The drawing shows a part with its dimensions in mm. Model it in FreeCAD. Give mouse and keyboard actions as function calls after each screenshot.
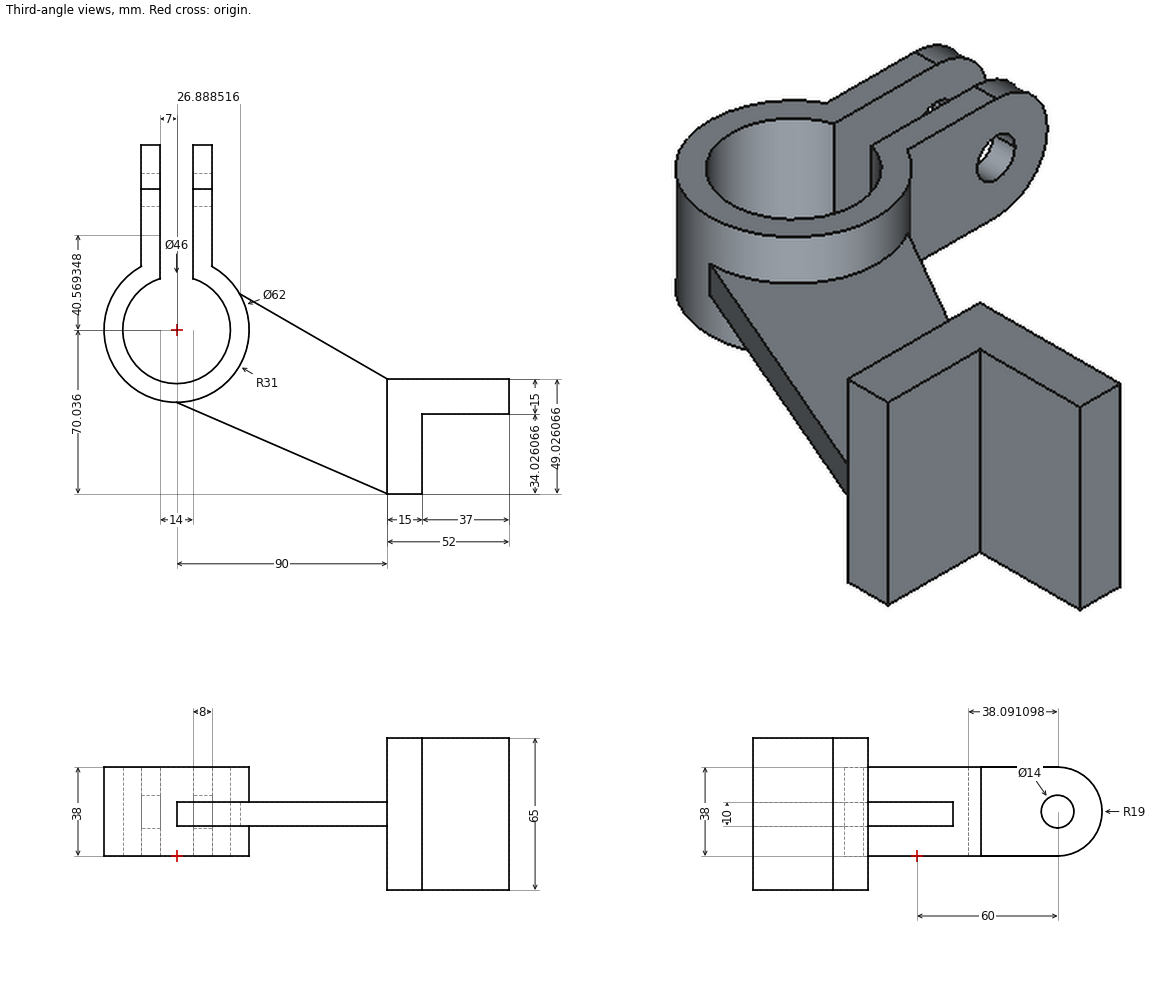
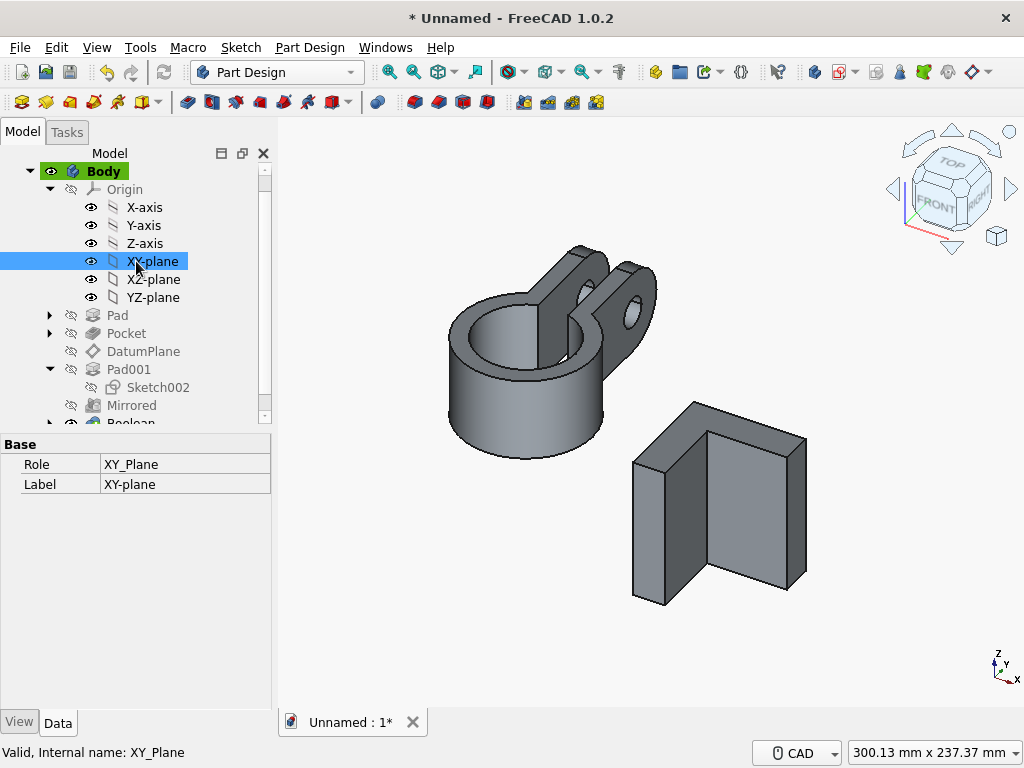
click(972, 72)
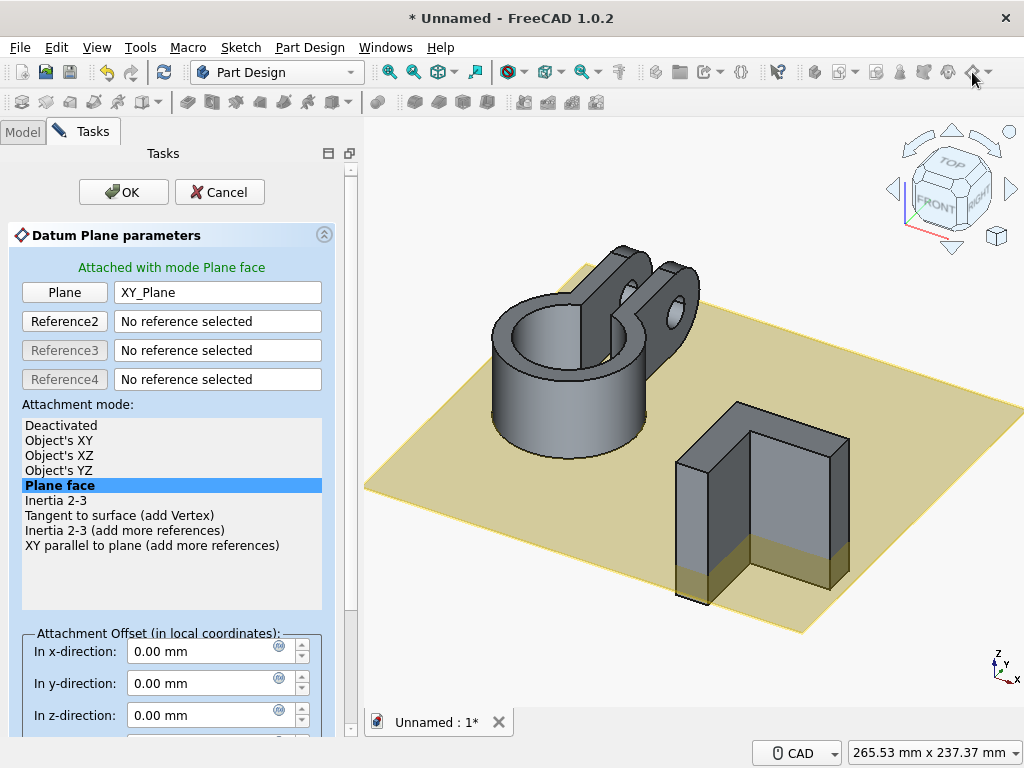
triple_click(210, 715)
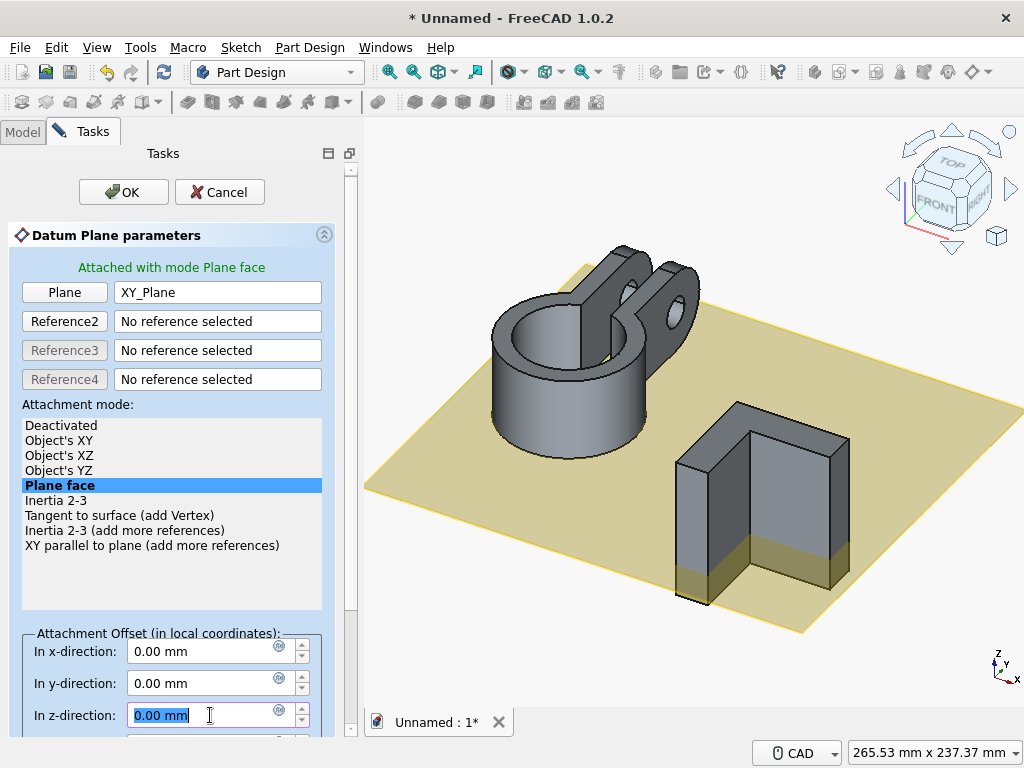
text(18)
key(Tab)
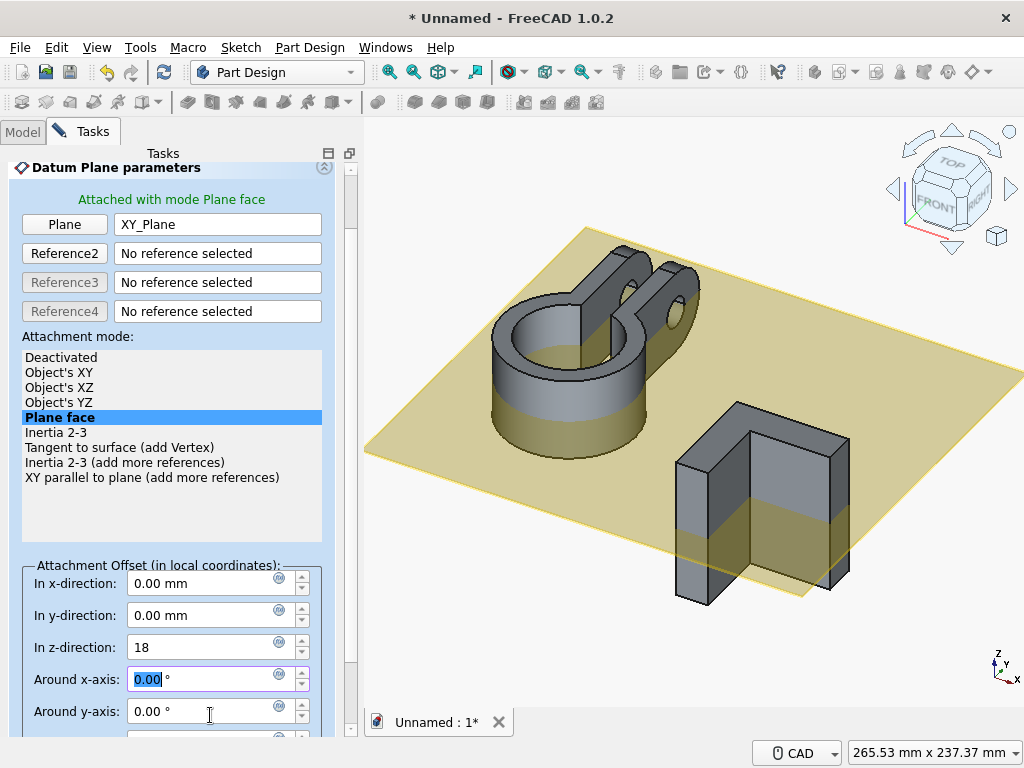
scroll(351, 450, up, 2)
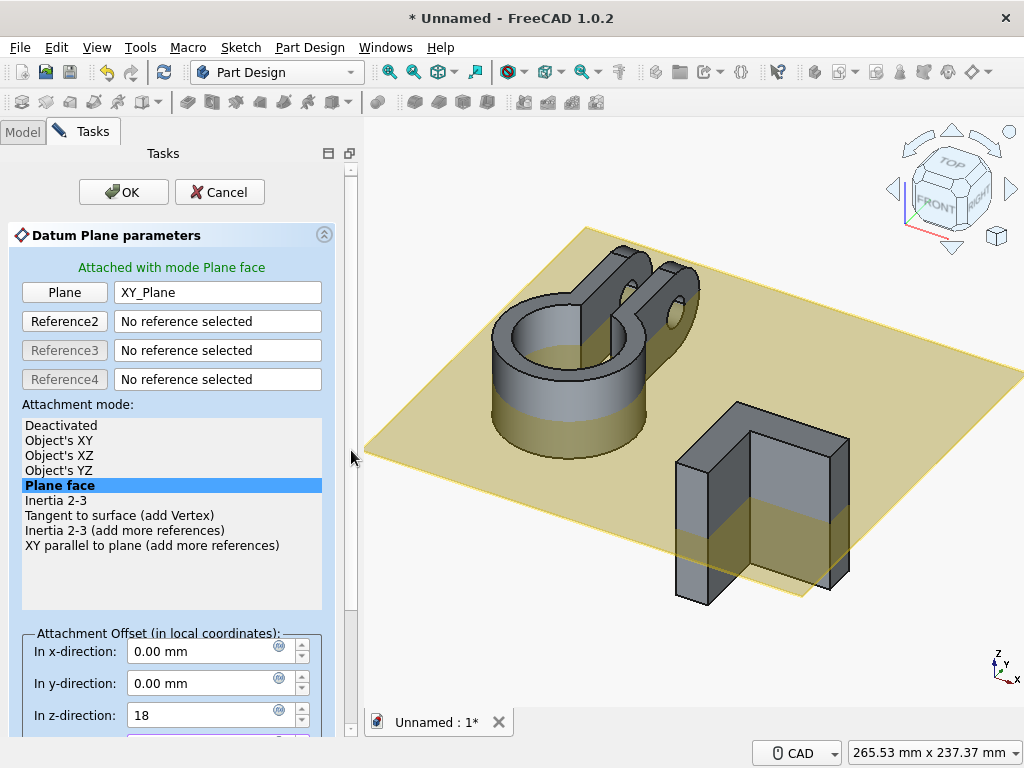
click(124, 192)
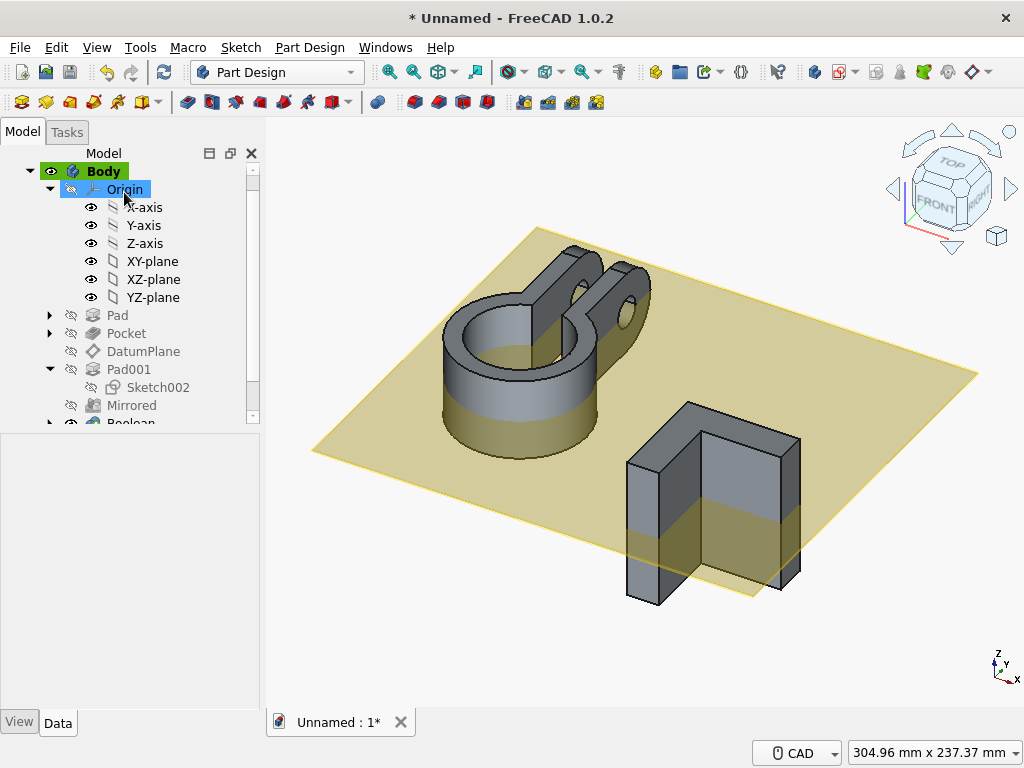
scroll(120, 293, down, 3)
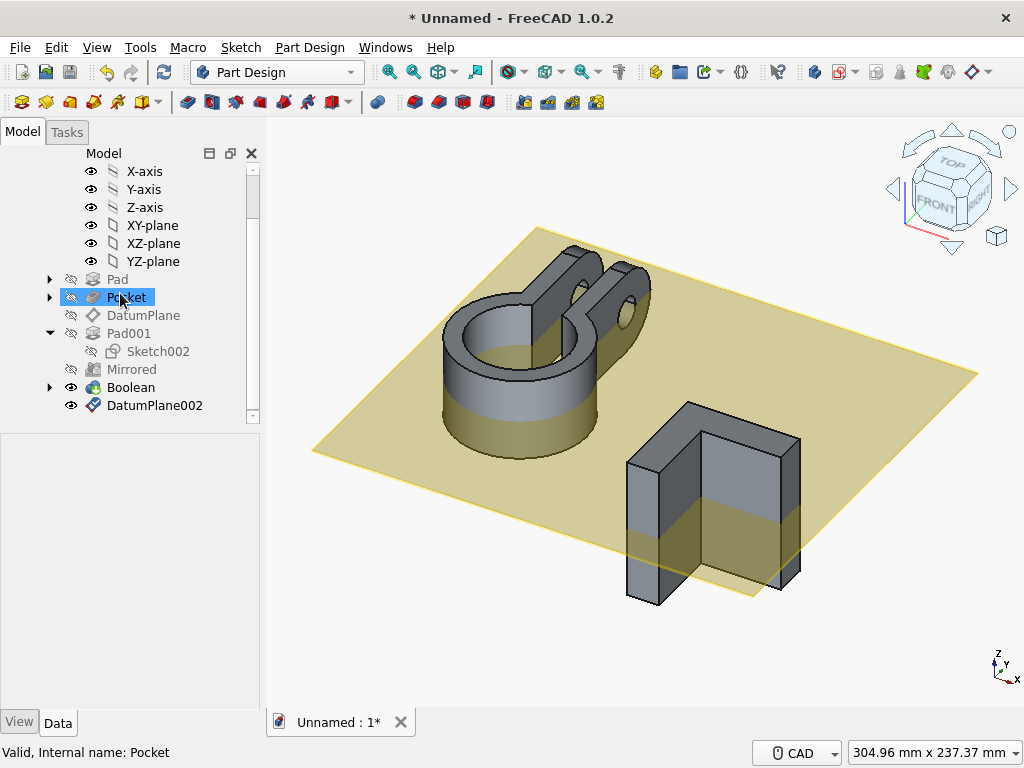
click(116, 405)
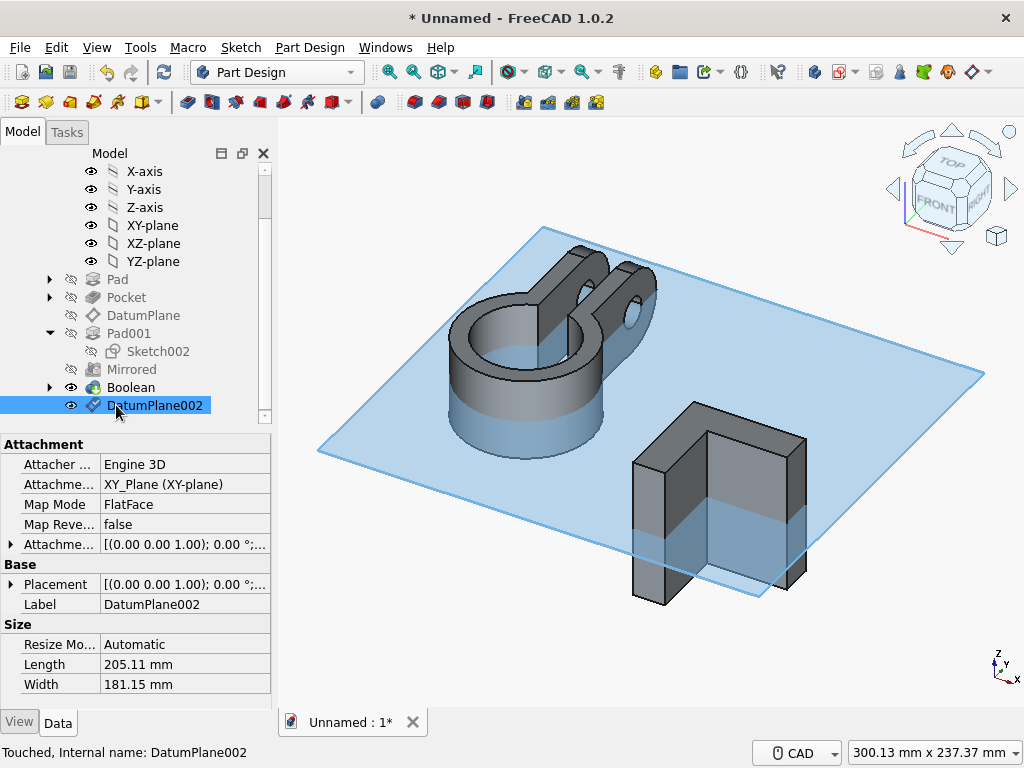
click(840, 72)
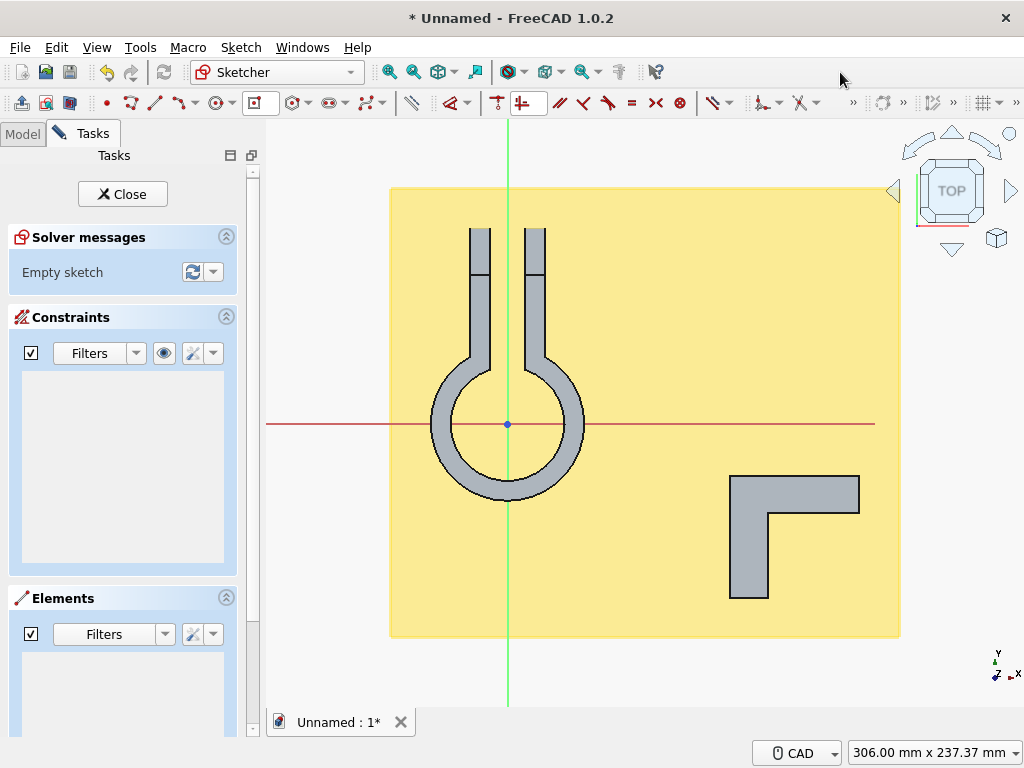
click(70, 104)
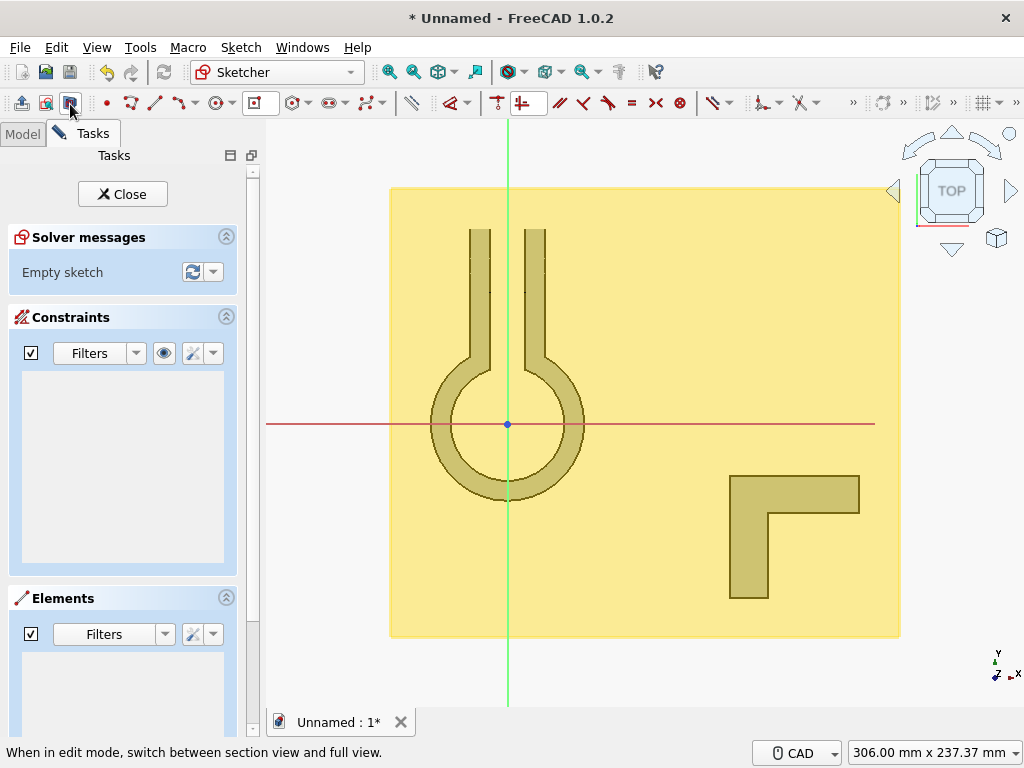
scroll(294, 147, down, 1)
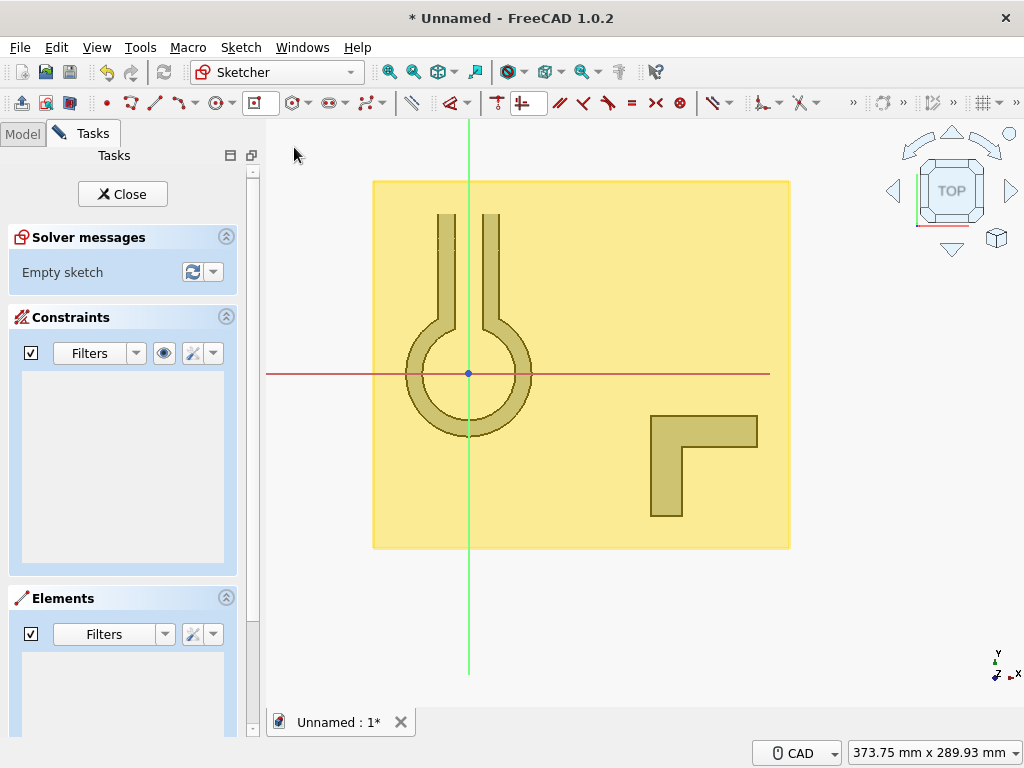
scroll(687, 462, up, 2)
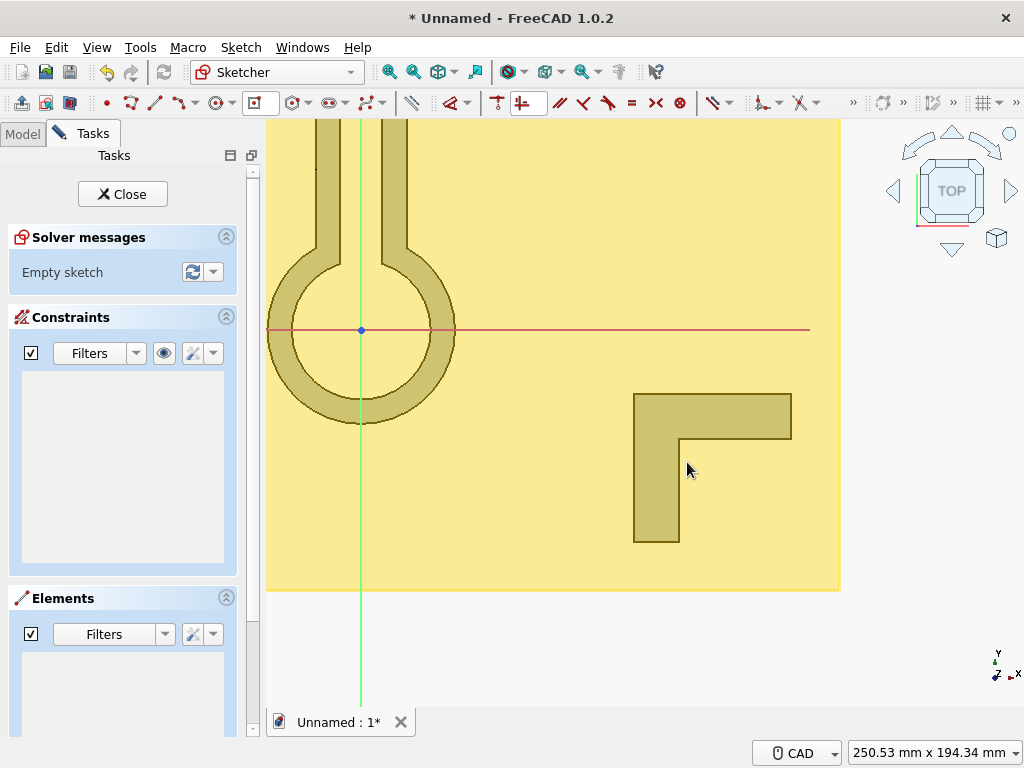
click(132, 104)